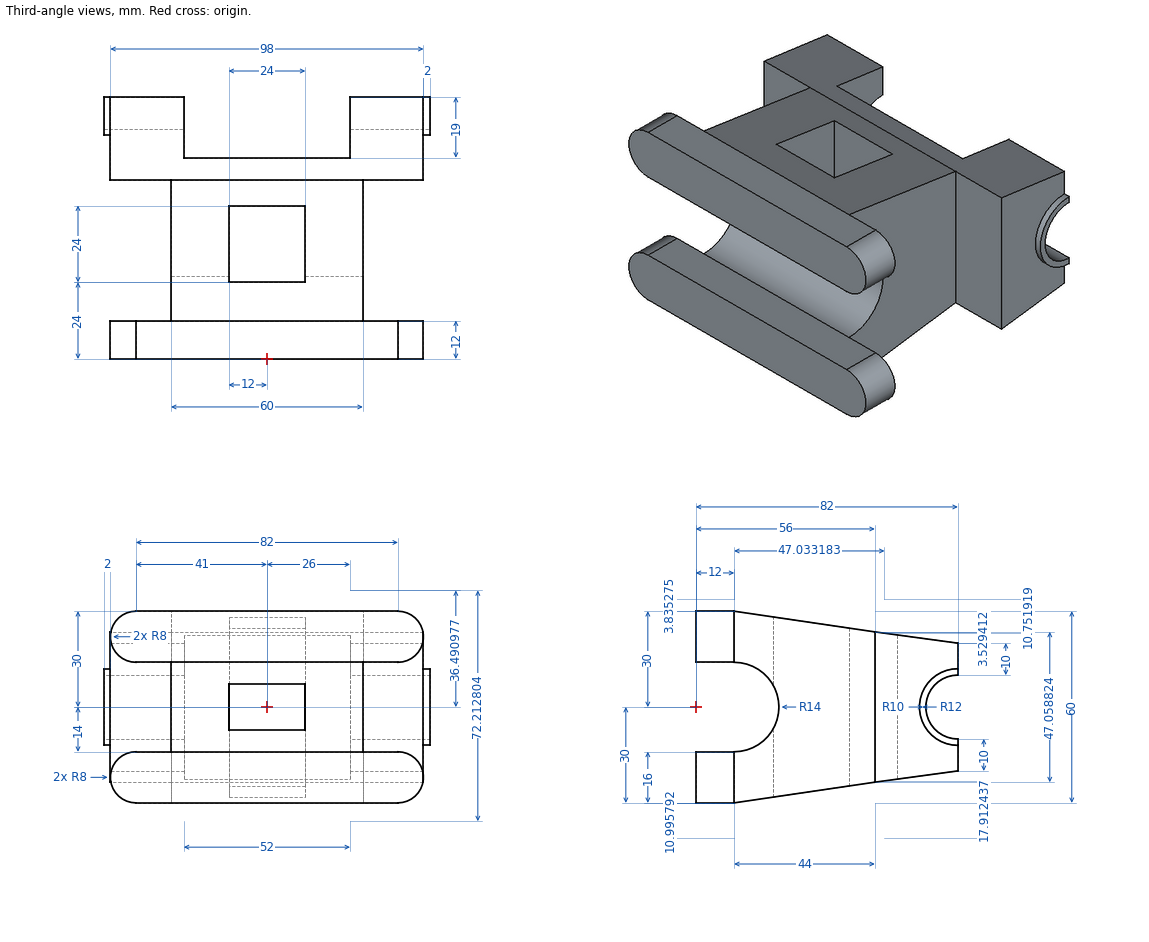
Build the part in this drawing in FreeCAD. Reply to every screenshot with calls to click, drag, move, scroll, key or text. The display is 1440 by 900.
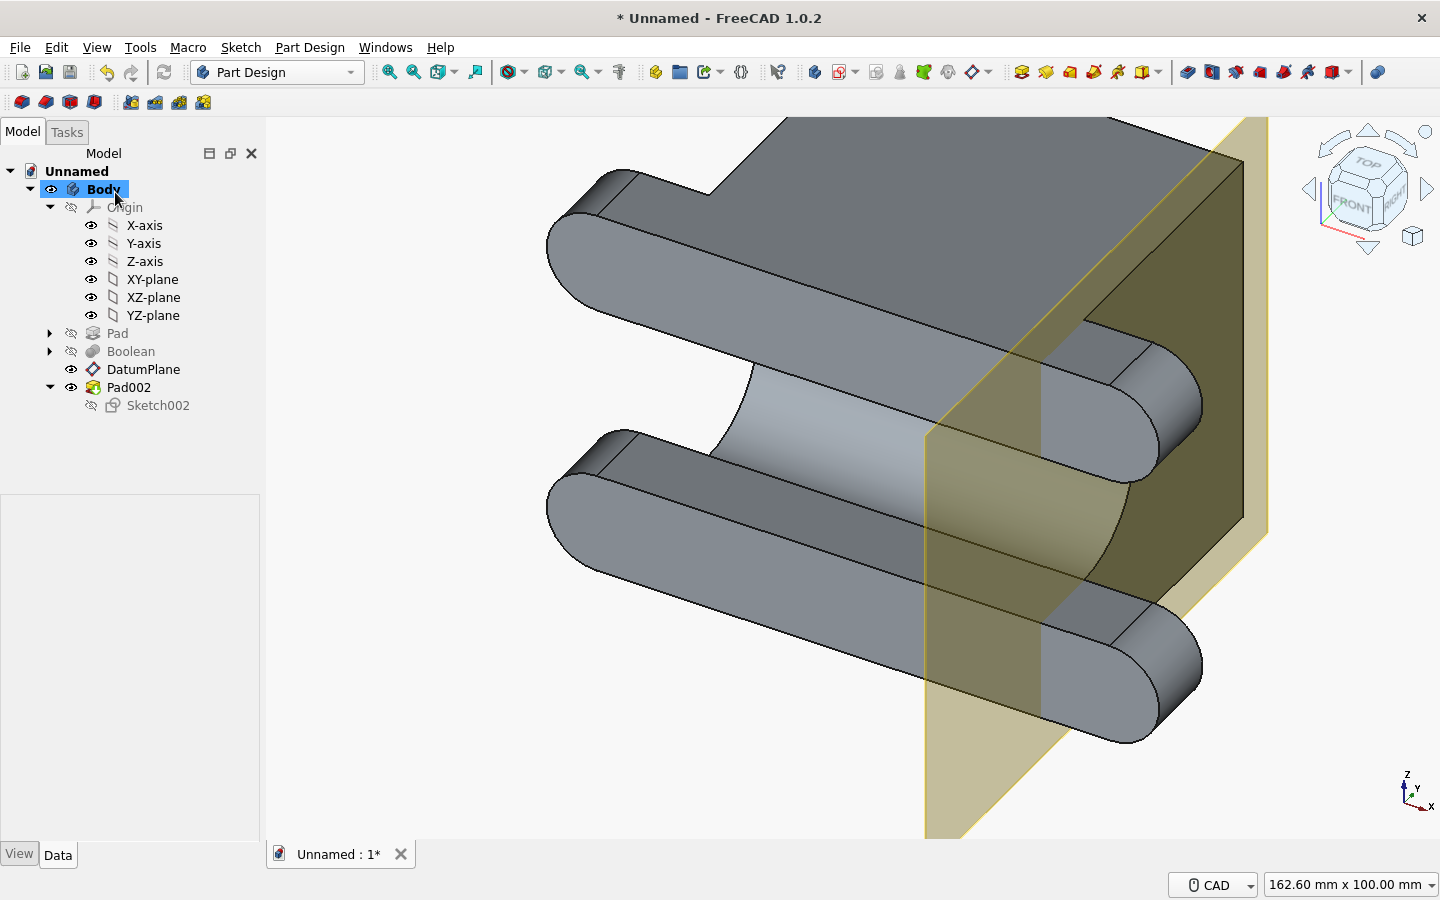
click(116, 369)
key(space)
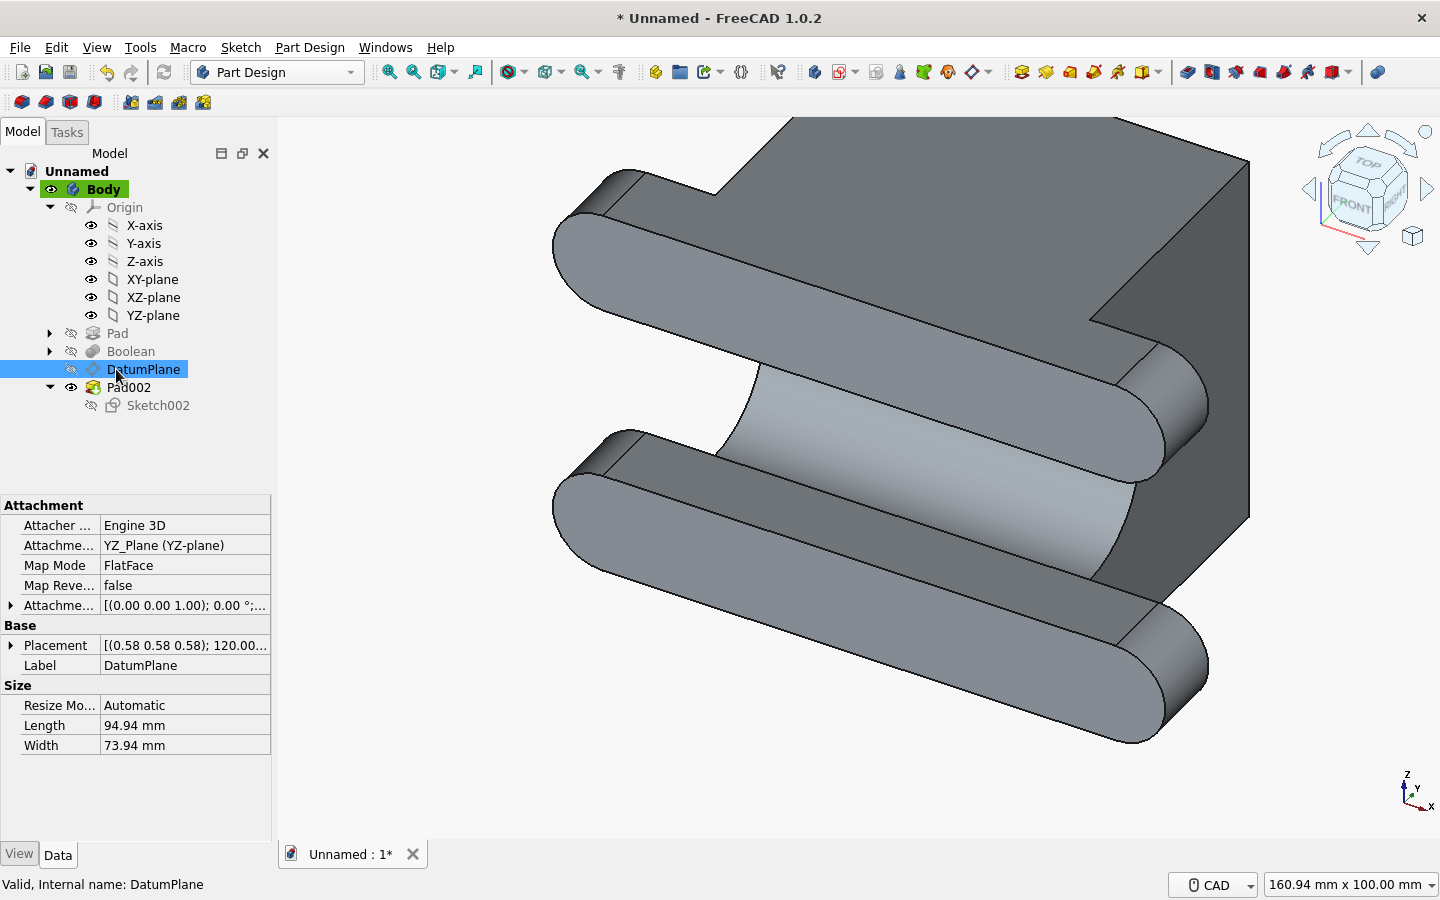
click(390, 72)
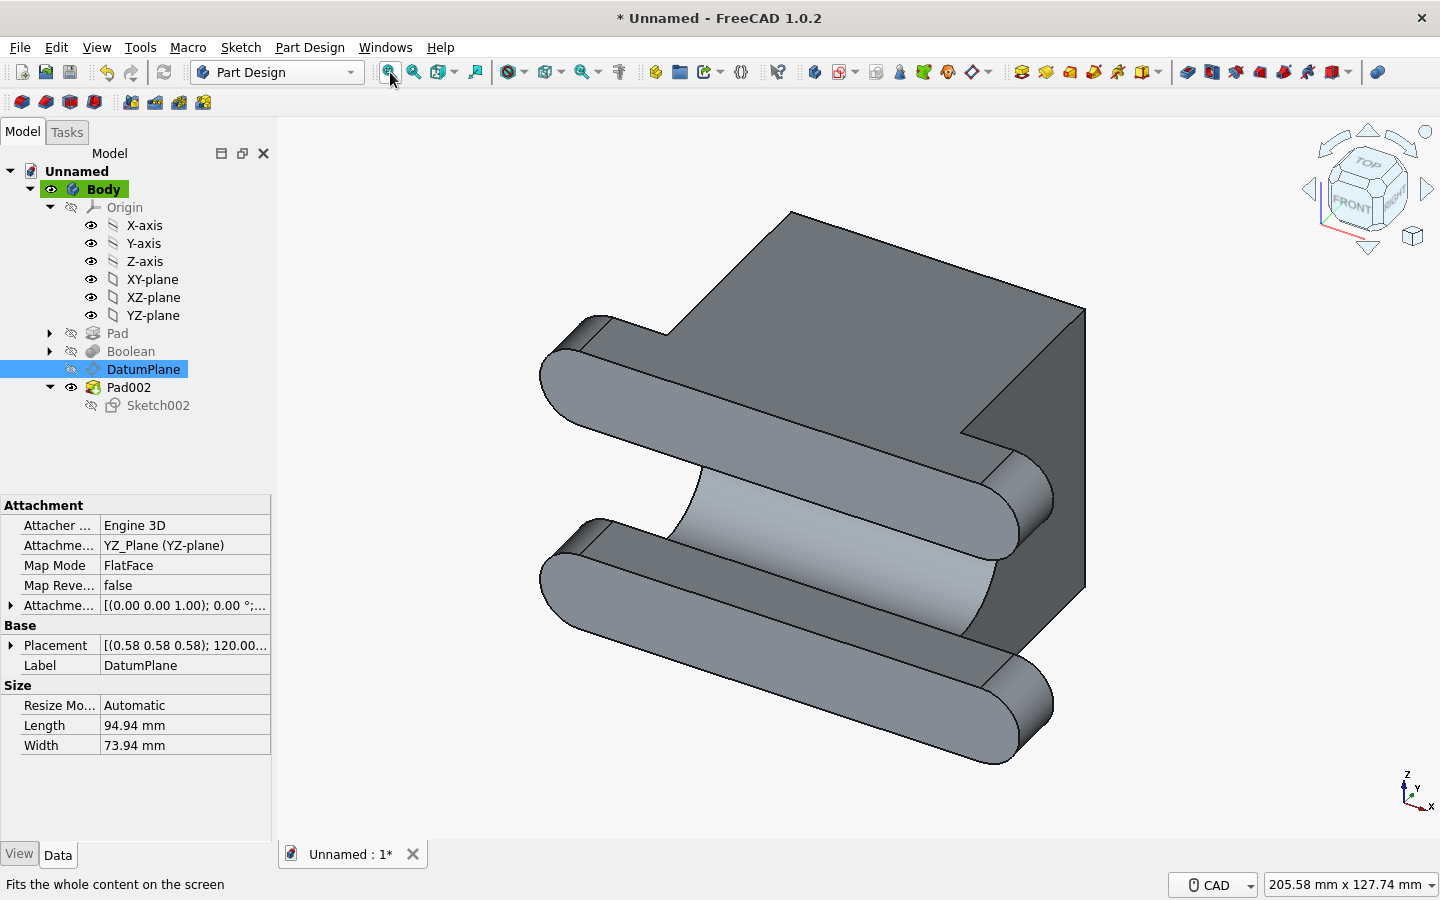
click(1041, 451)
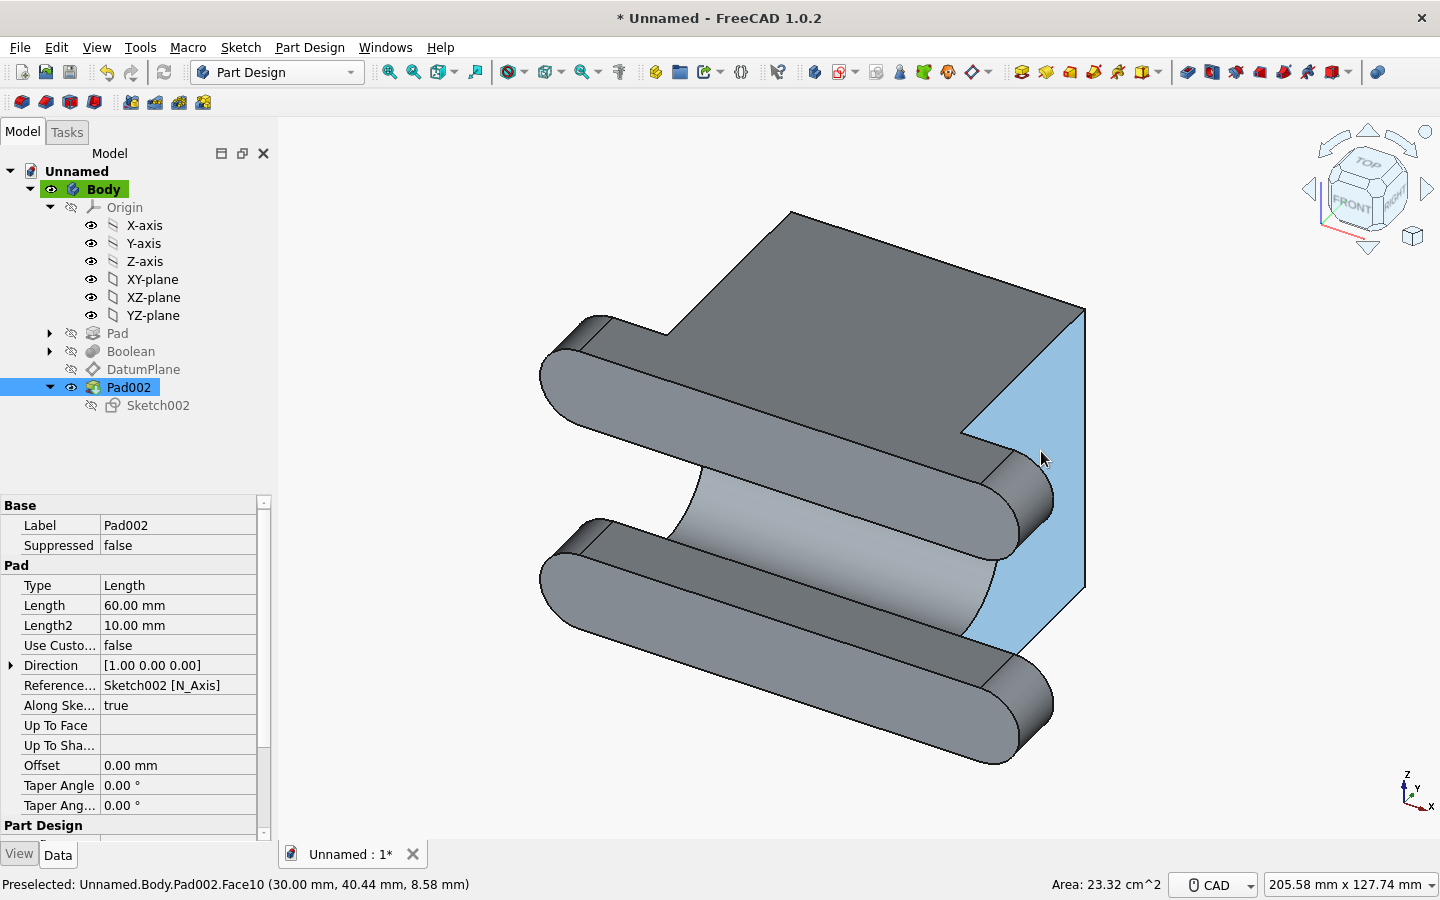
click(840, 72)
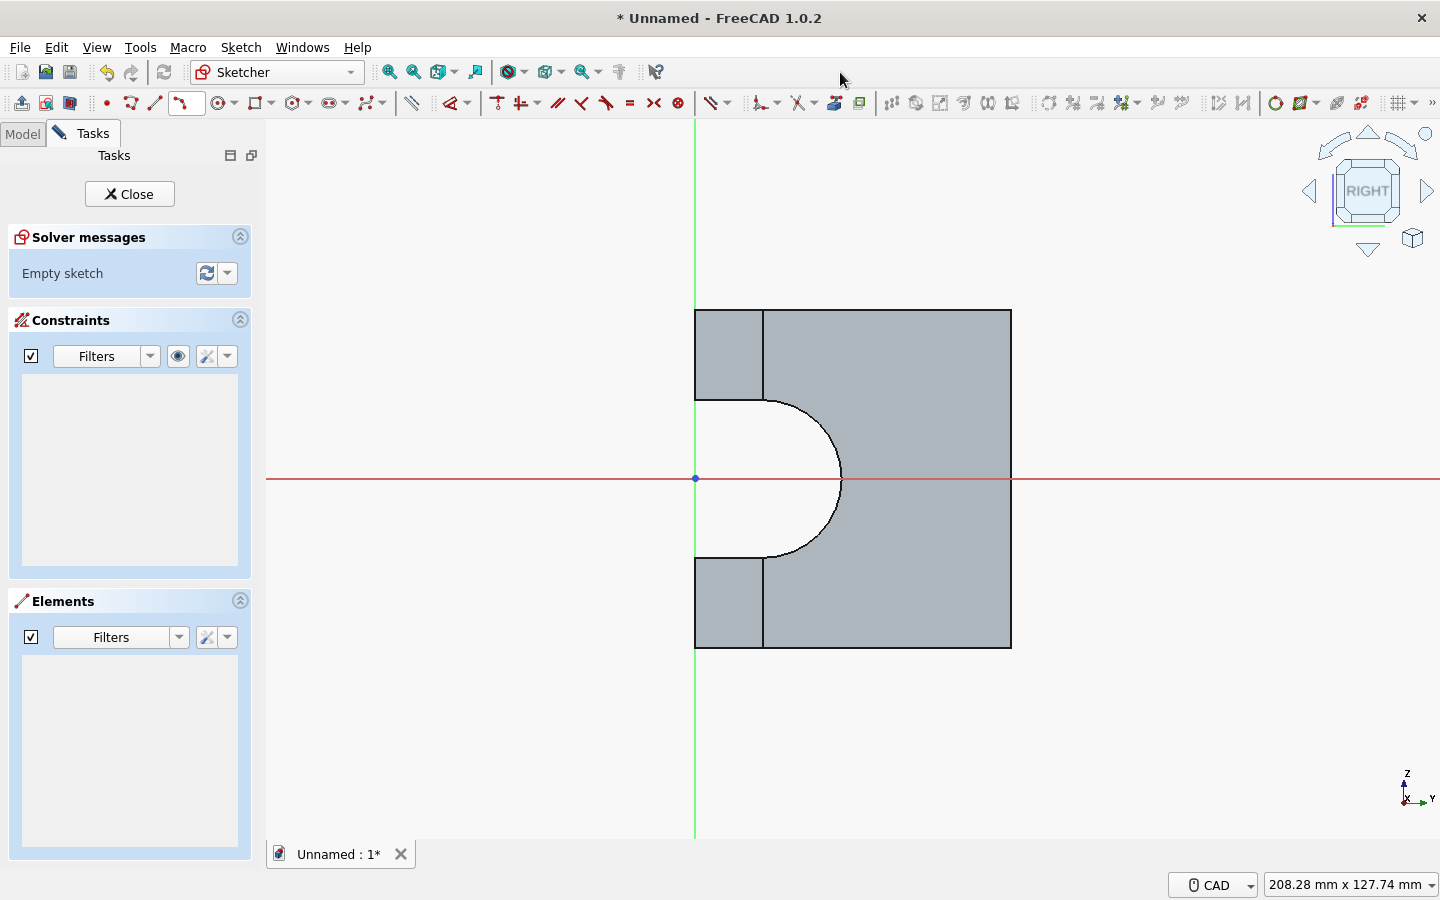
click(132, 104)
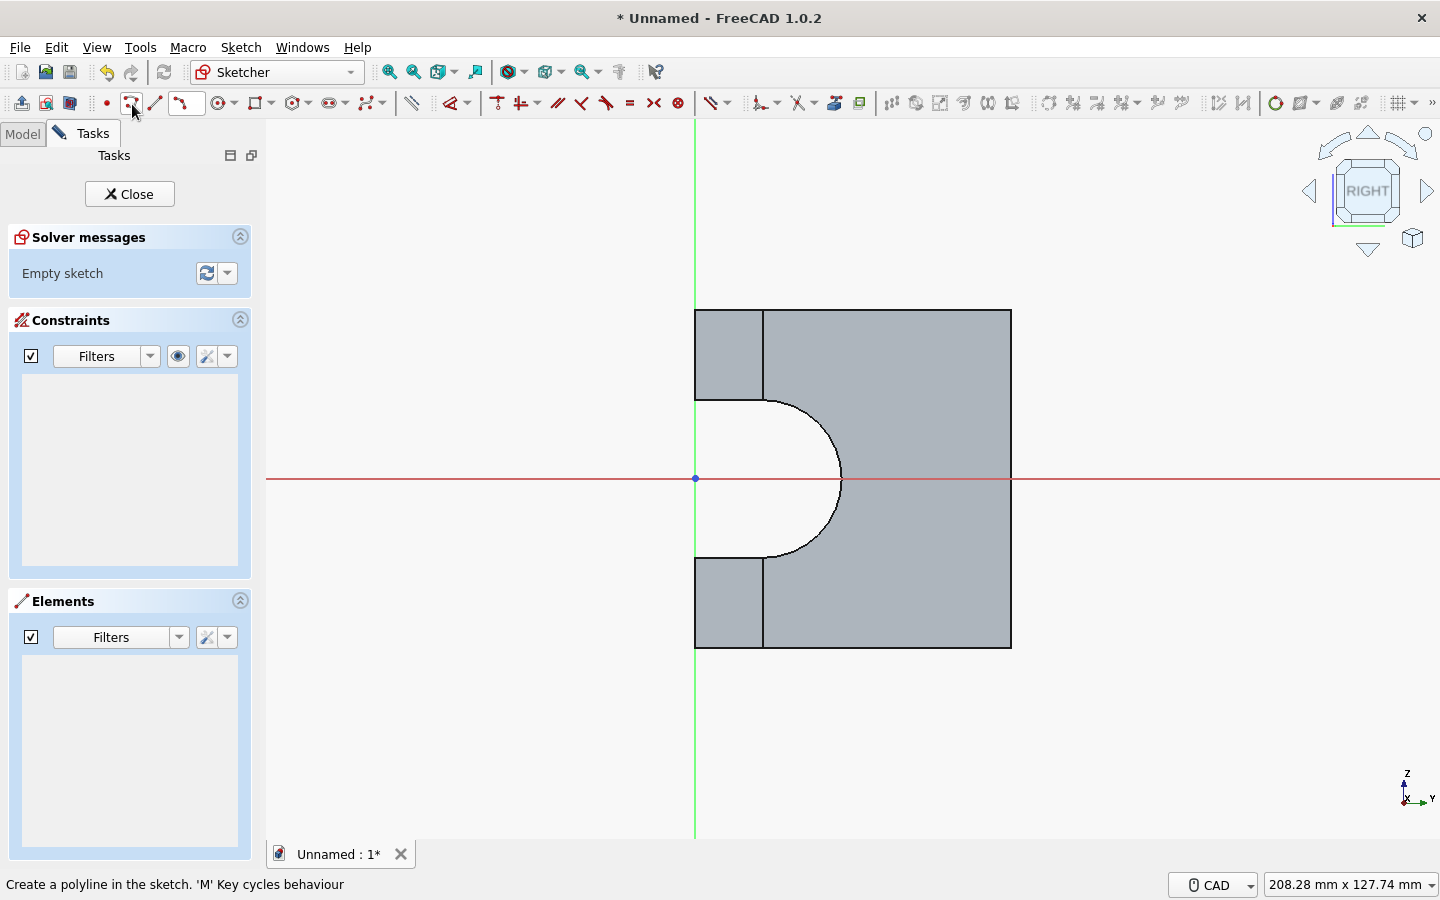
click(763, 310)
click(1028, 349)
click(1028, 288)
click(763, 288)
click(763, 311)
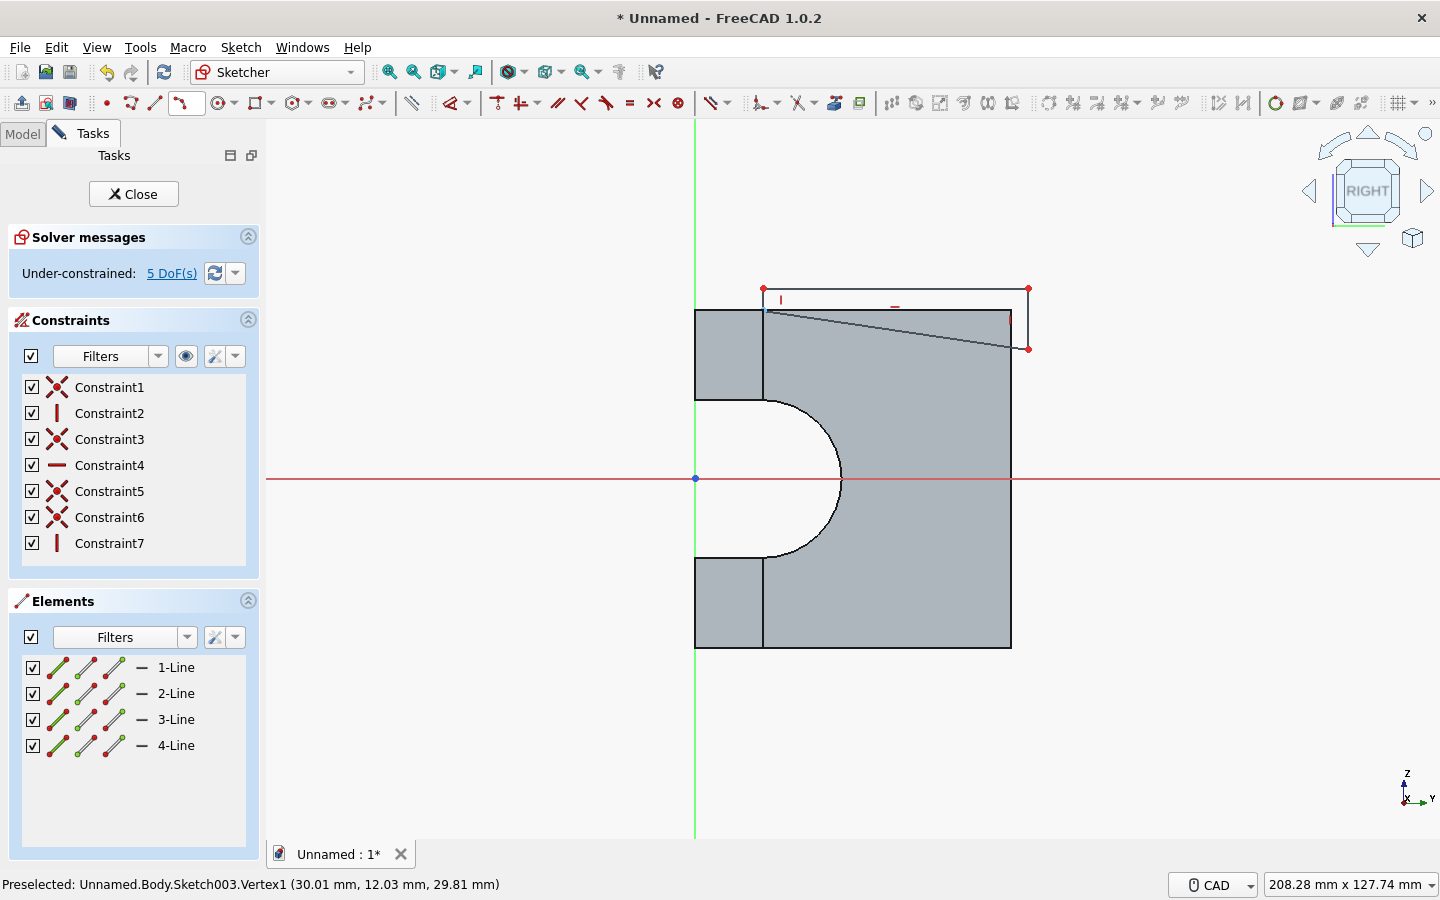
click(763, 648)
click(763, 710)
click(1028, 710)
click(1028, 609)
click(763, 649)
key(Escape)
key(Escape)